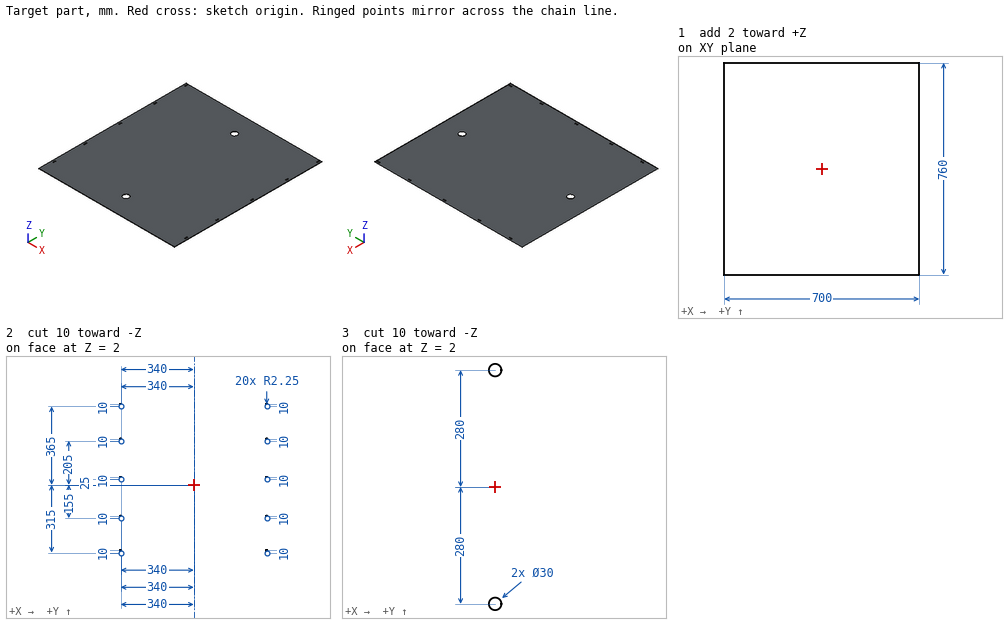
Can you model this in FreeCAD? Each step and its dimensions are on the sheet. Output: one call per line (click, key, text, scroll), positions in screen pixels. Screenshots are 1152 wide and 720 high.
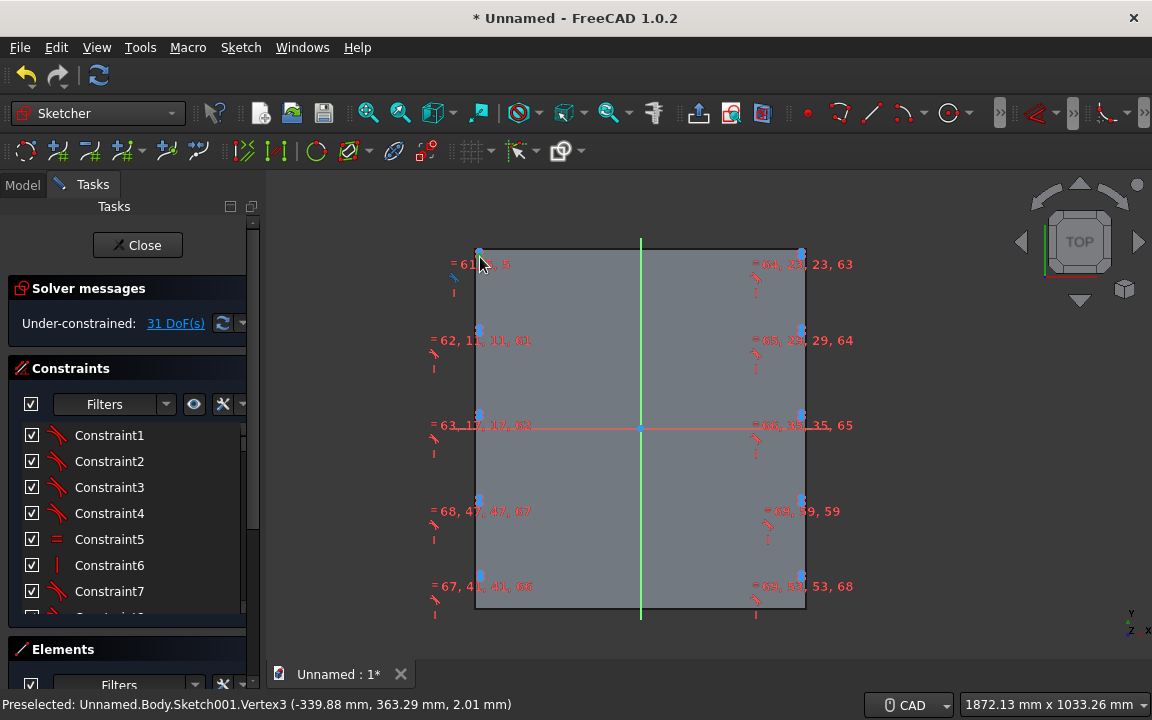
scroll(802, 257, up, 13)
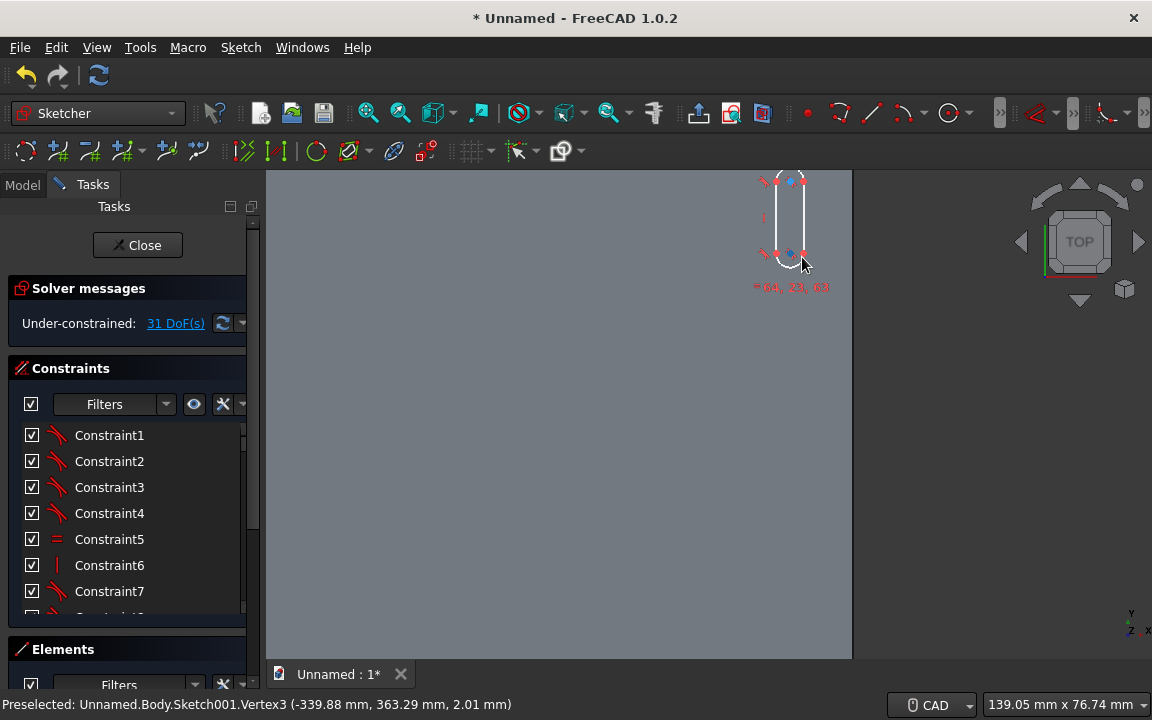
click(790, 254)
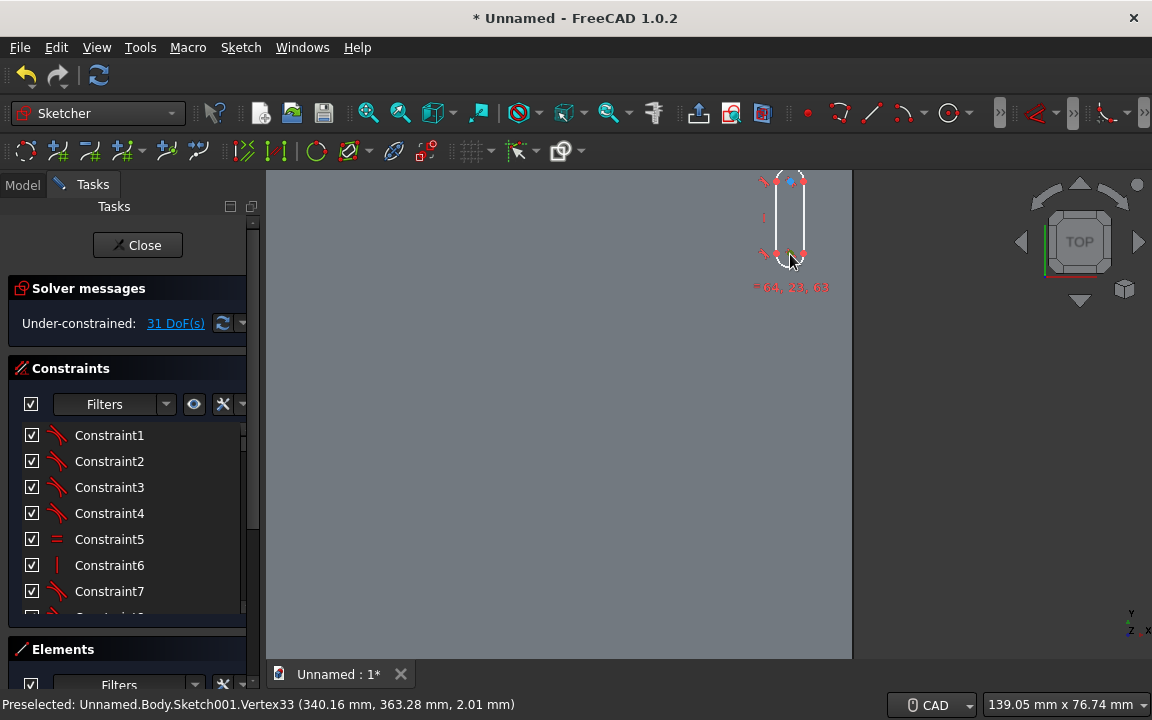
scroll(802, 257, down, 13)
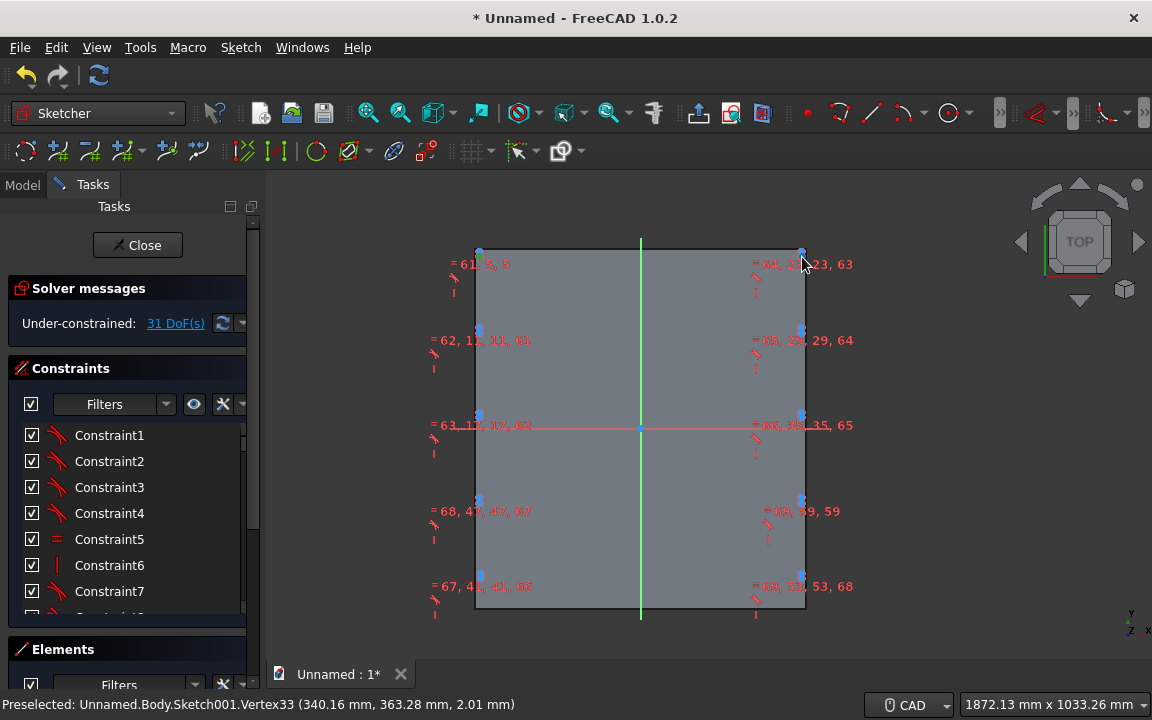
click(641, 600)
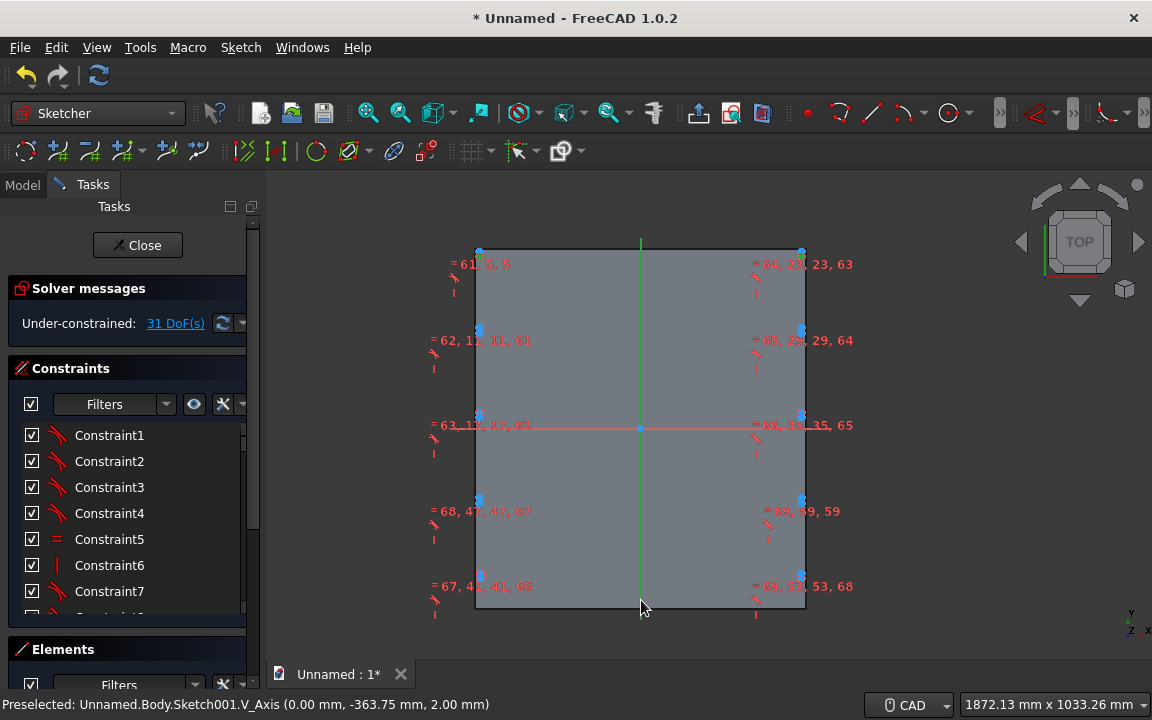
key(s)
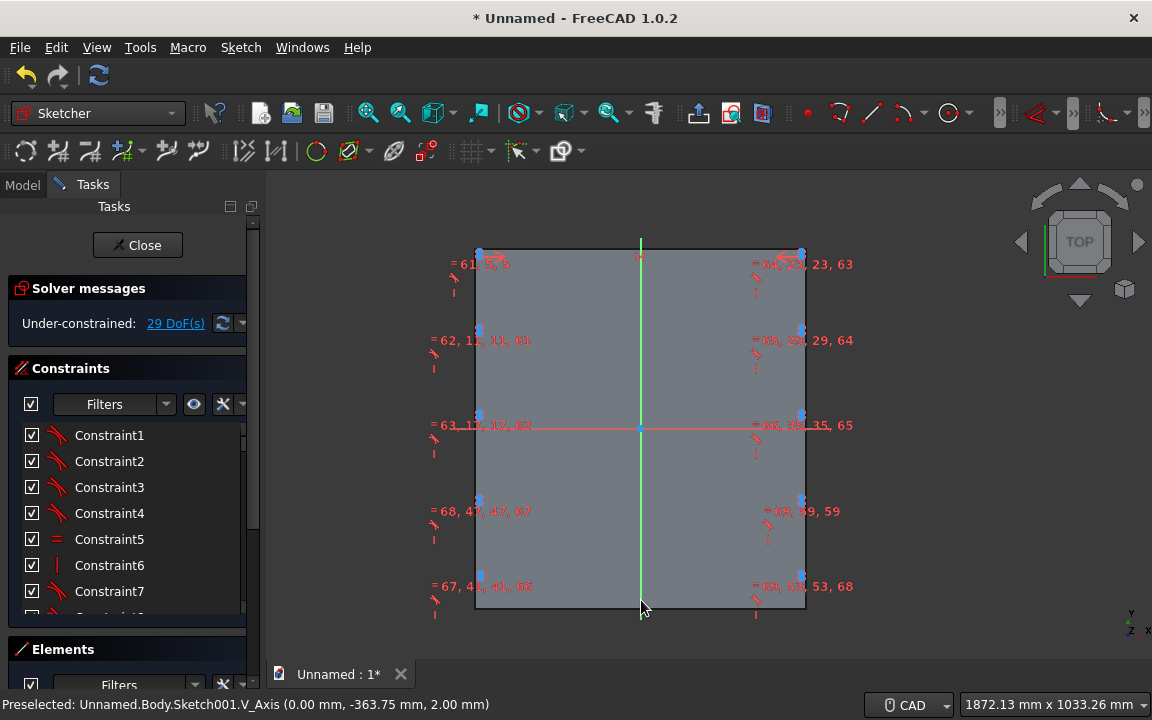
scroll(480, 333, up, 13)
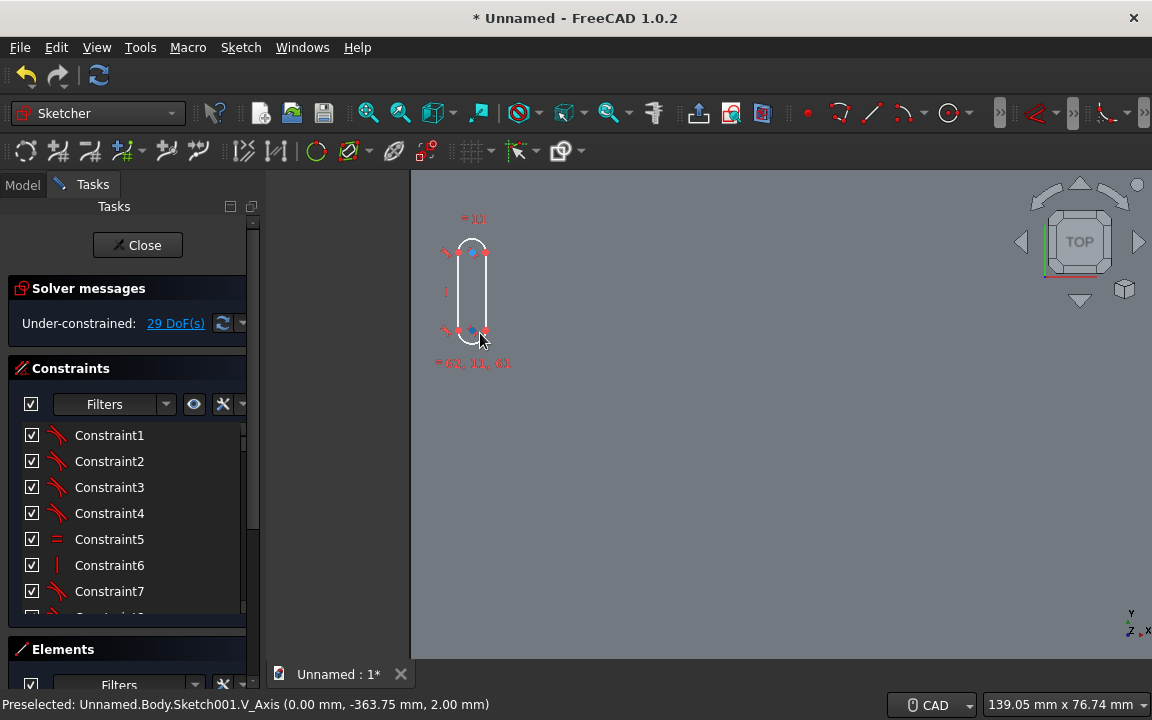
click(472, 330)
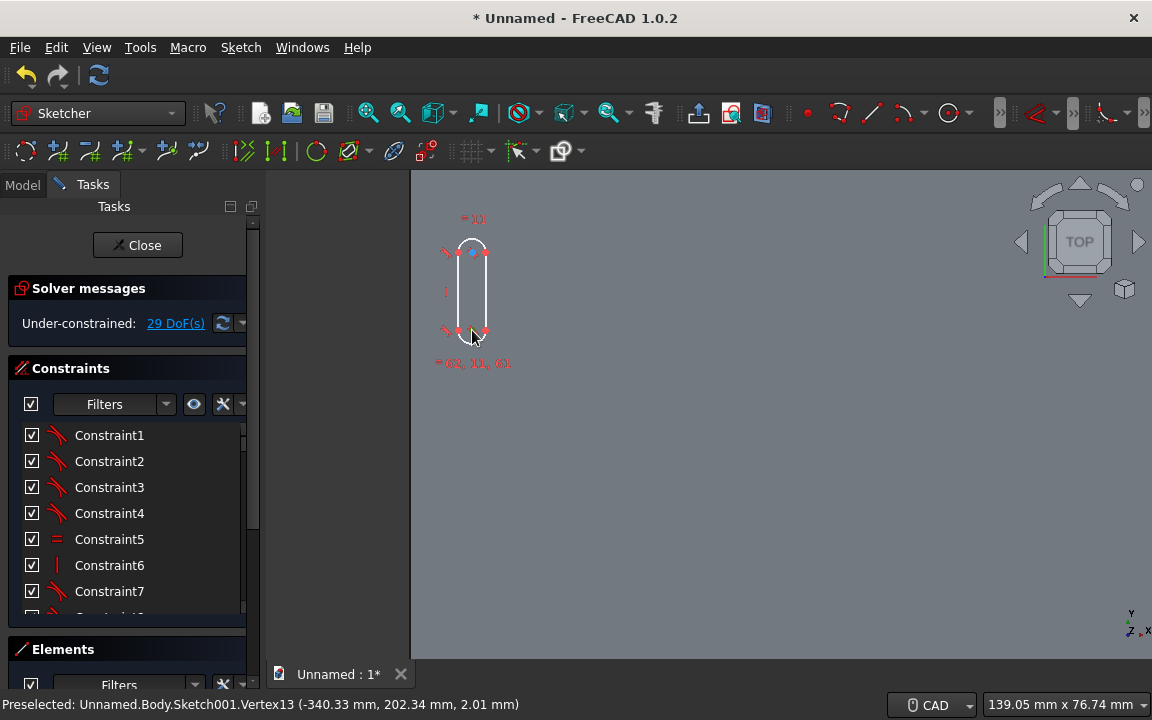
scroll(480, 333, down, 13)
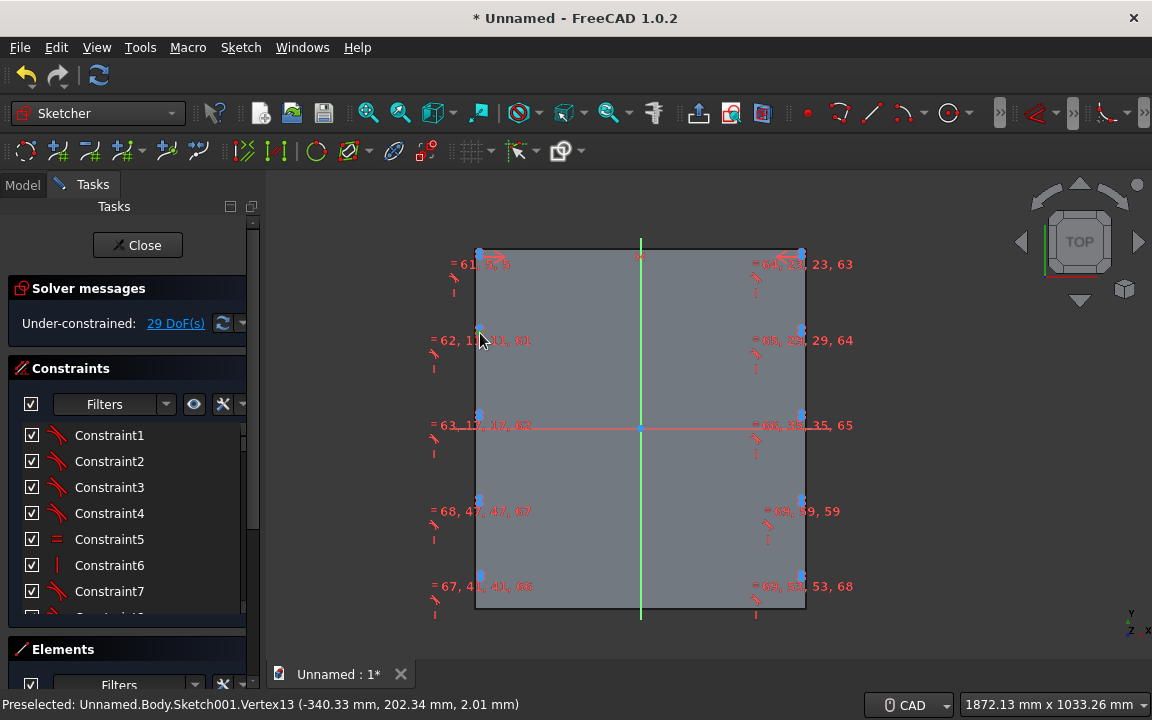
scroll(801, 333, up, 13)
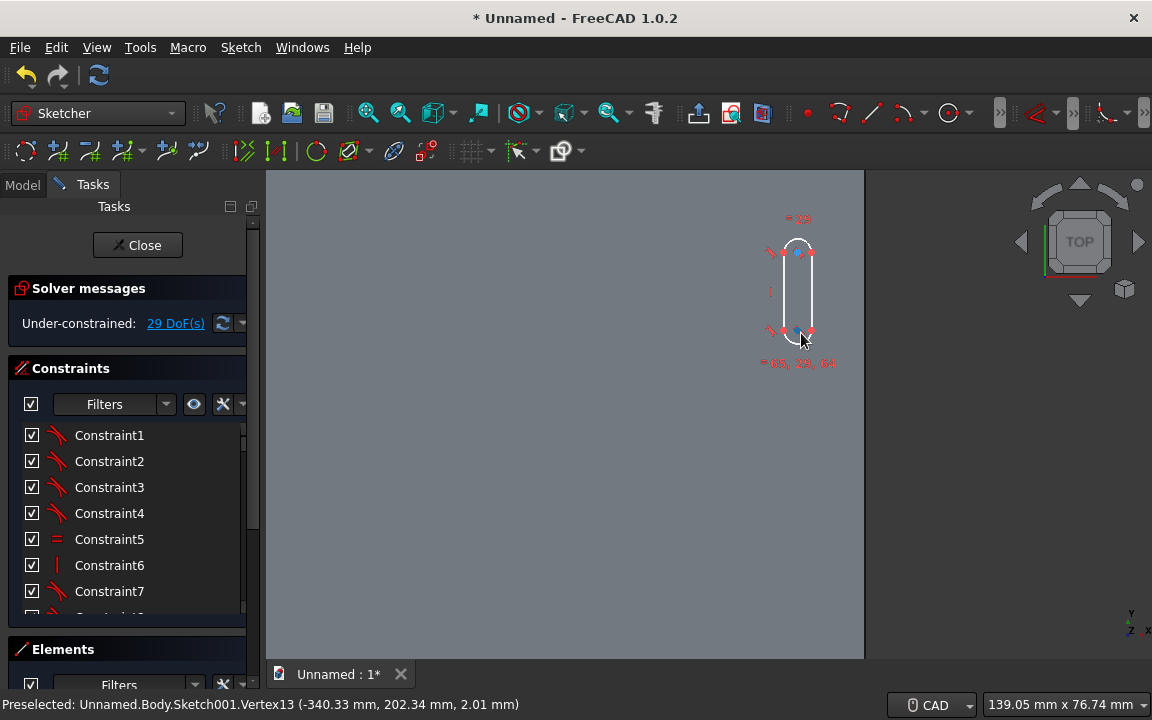
click(798, 330)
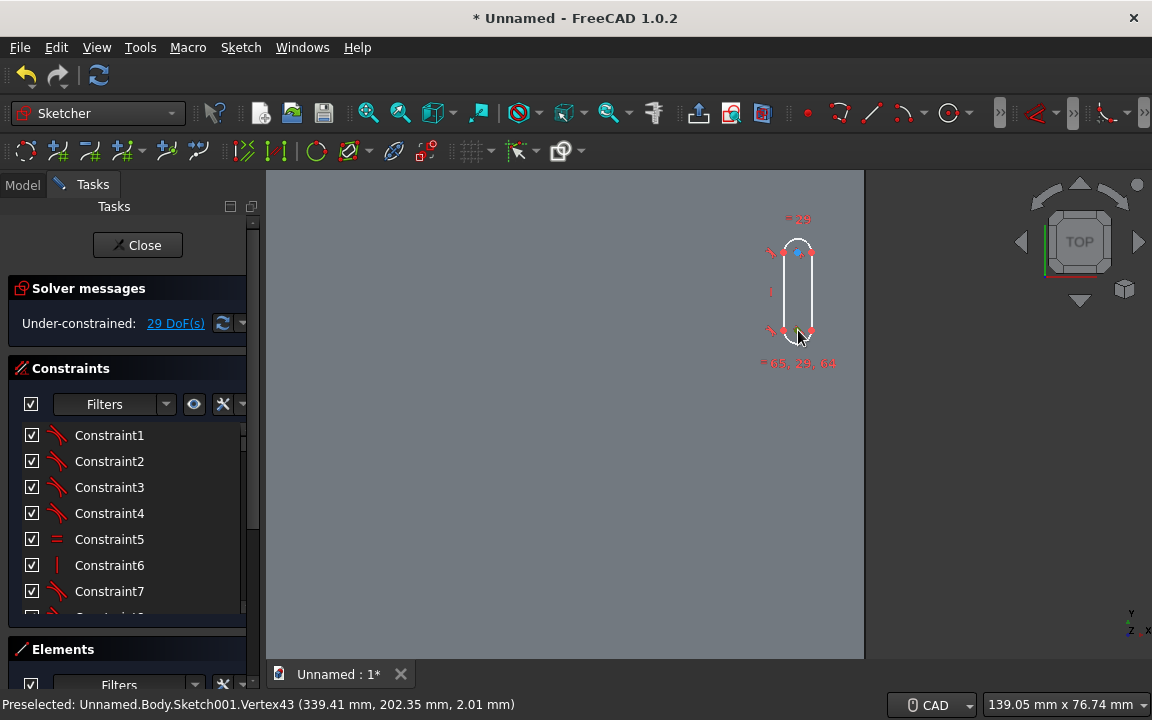
scroll(801, 333, down, 13)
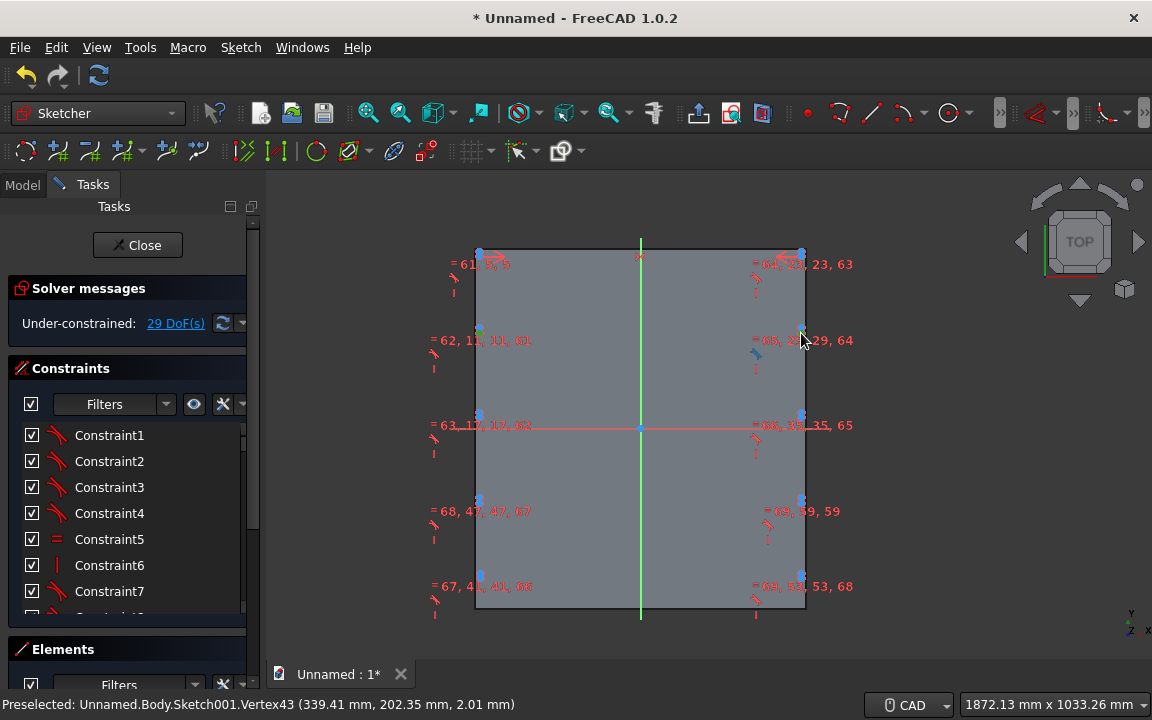
click(641, 600)